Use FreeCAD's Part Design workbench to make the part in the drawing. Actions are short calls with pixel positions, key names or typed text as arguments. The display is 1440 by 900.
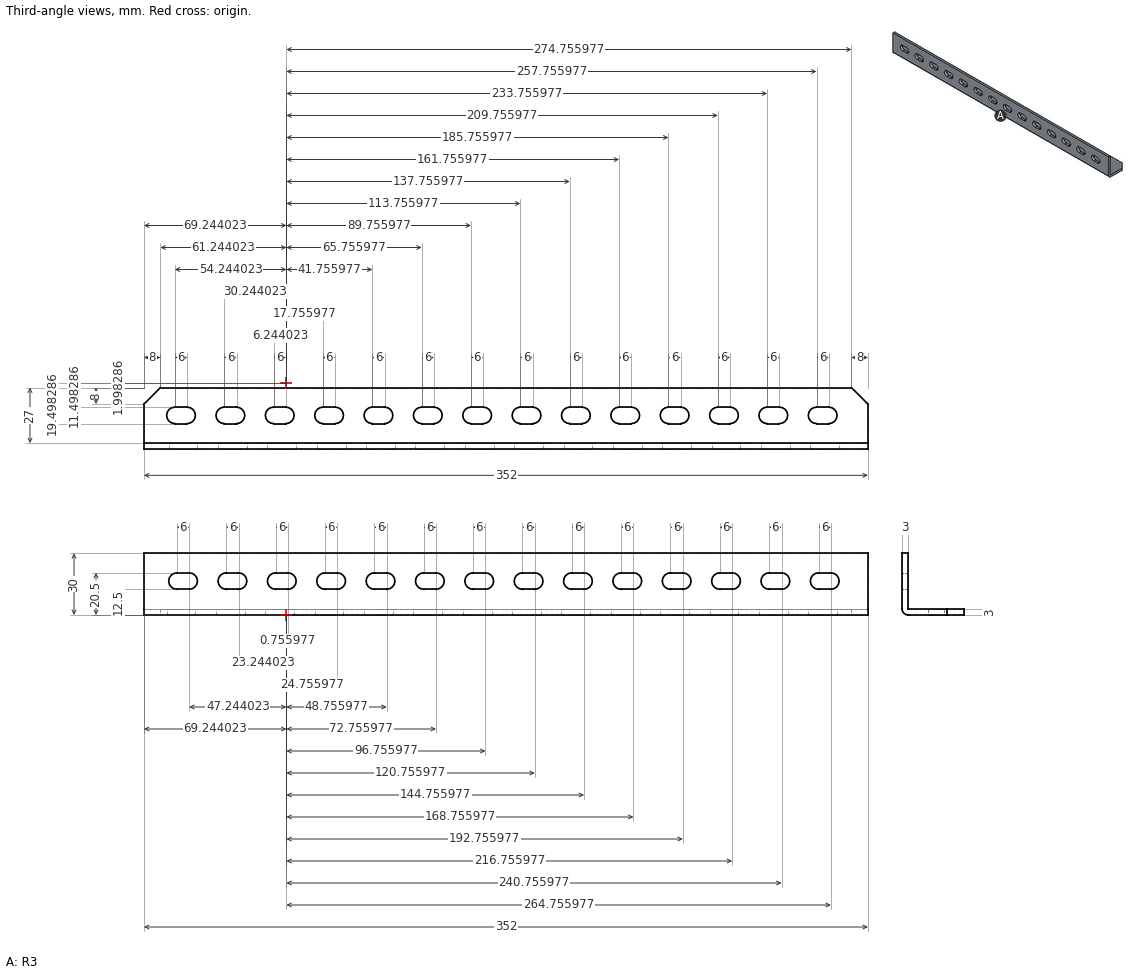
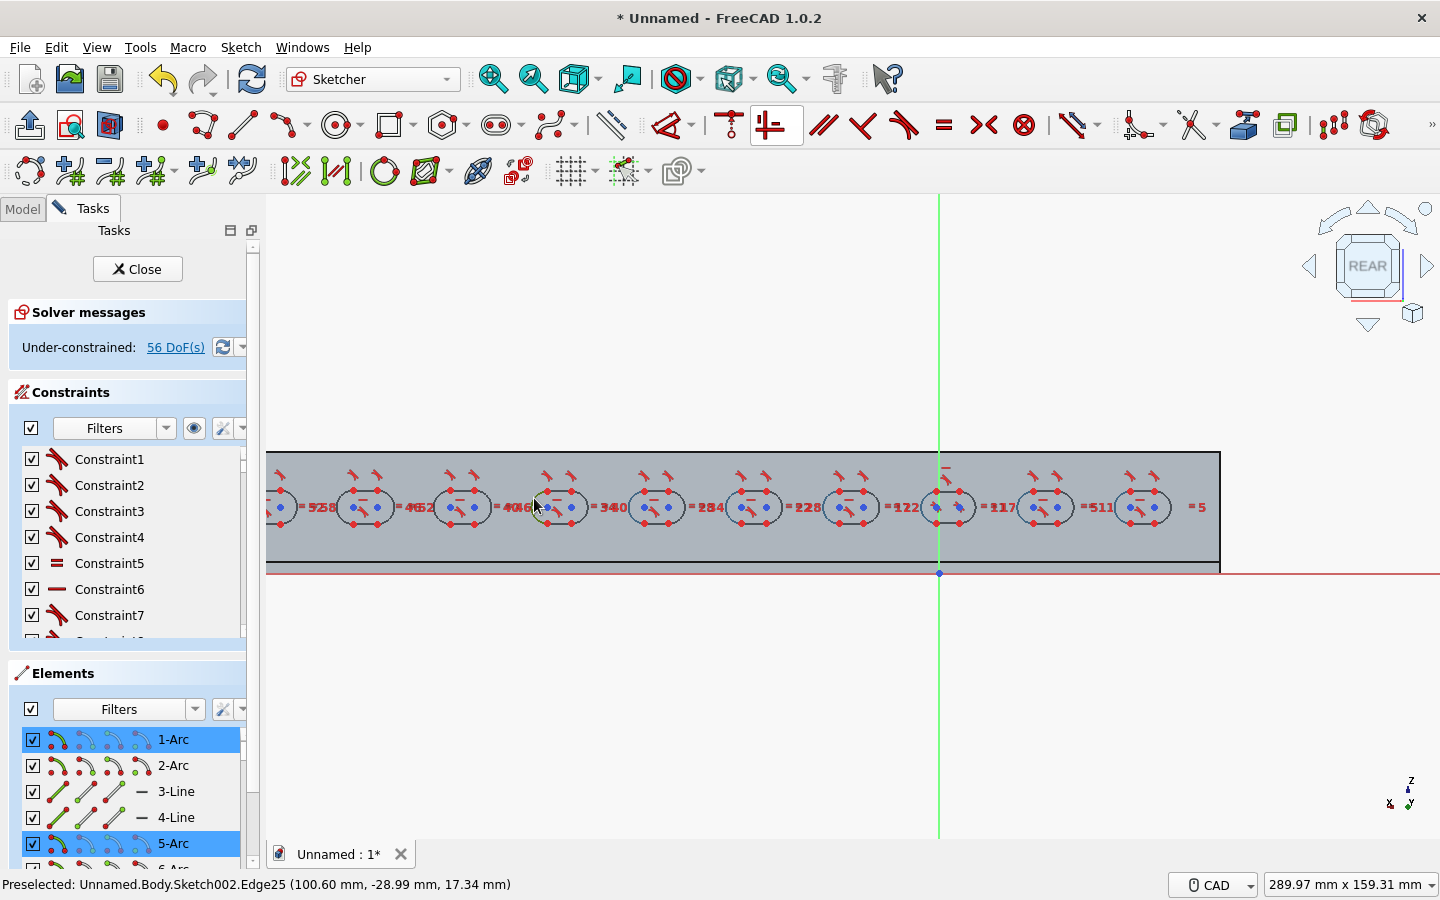
click(437, 497)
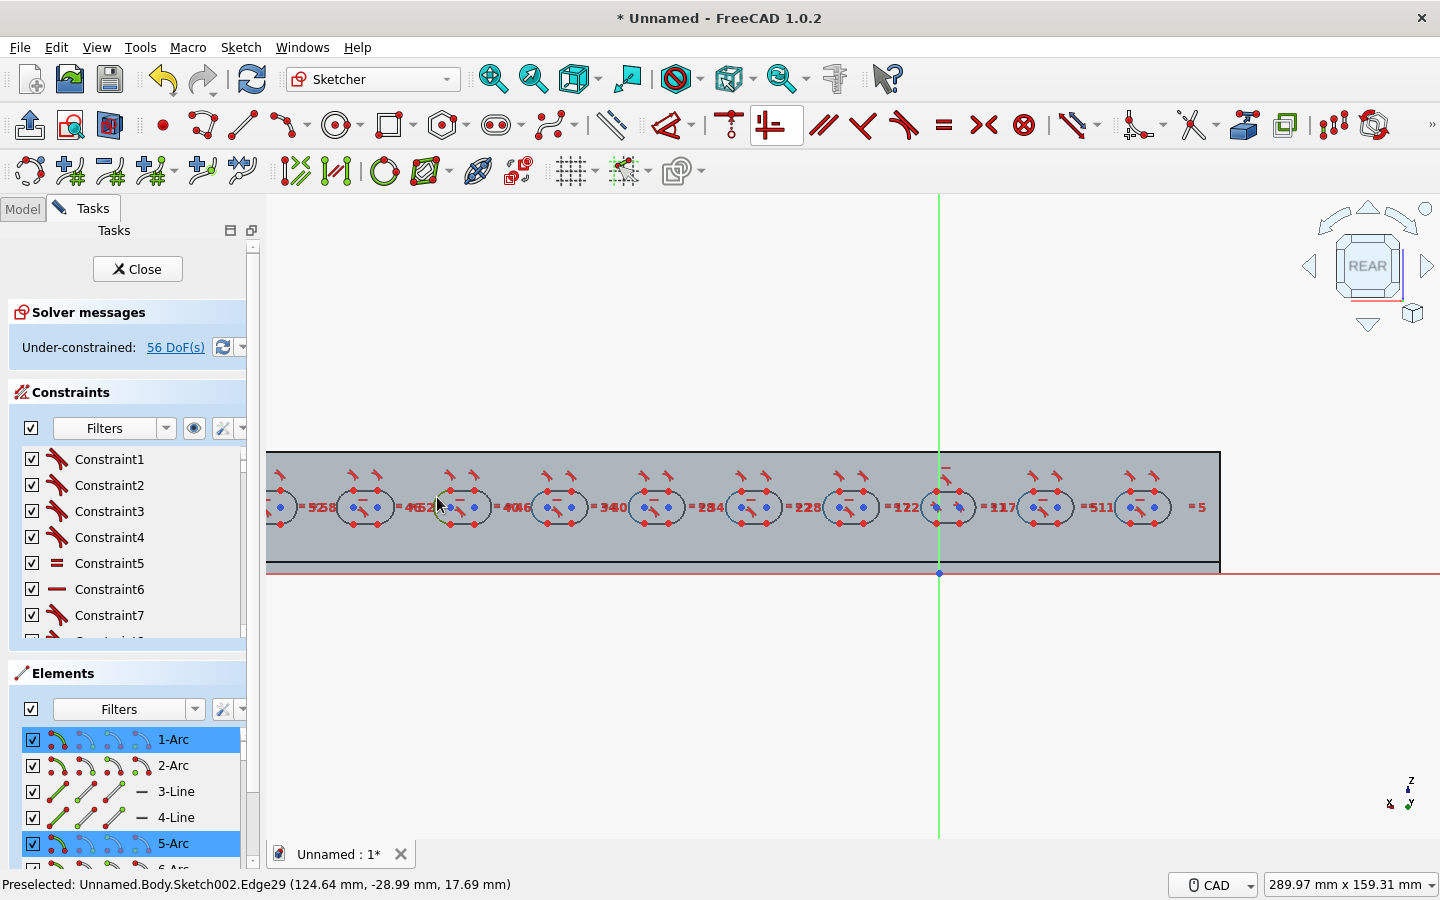
click(340, 497)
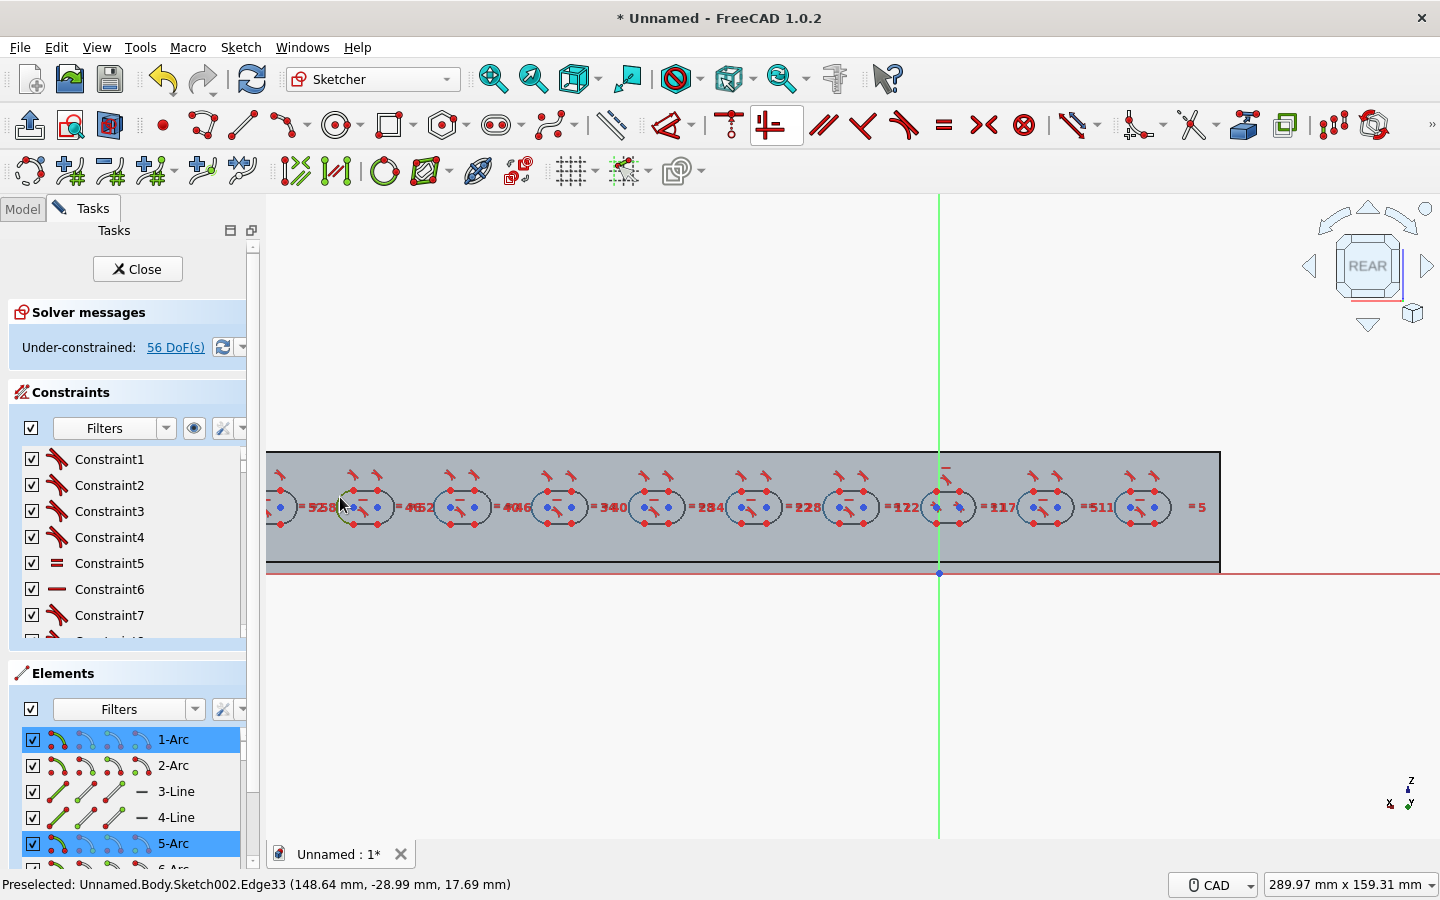
scroll(1117, 497, down, 3)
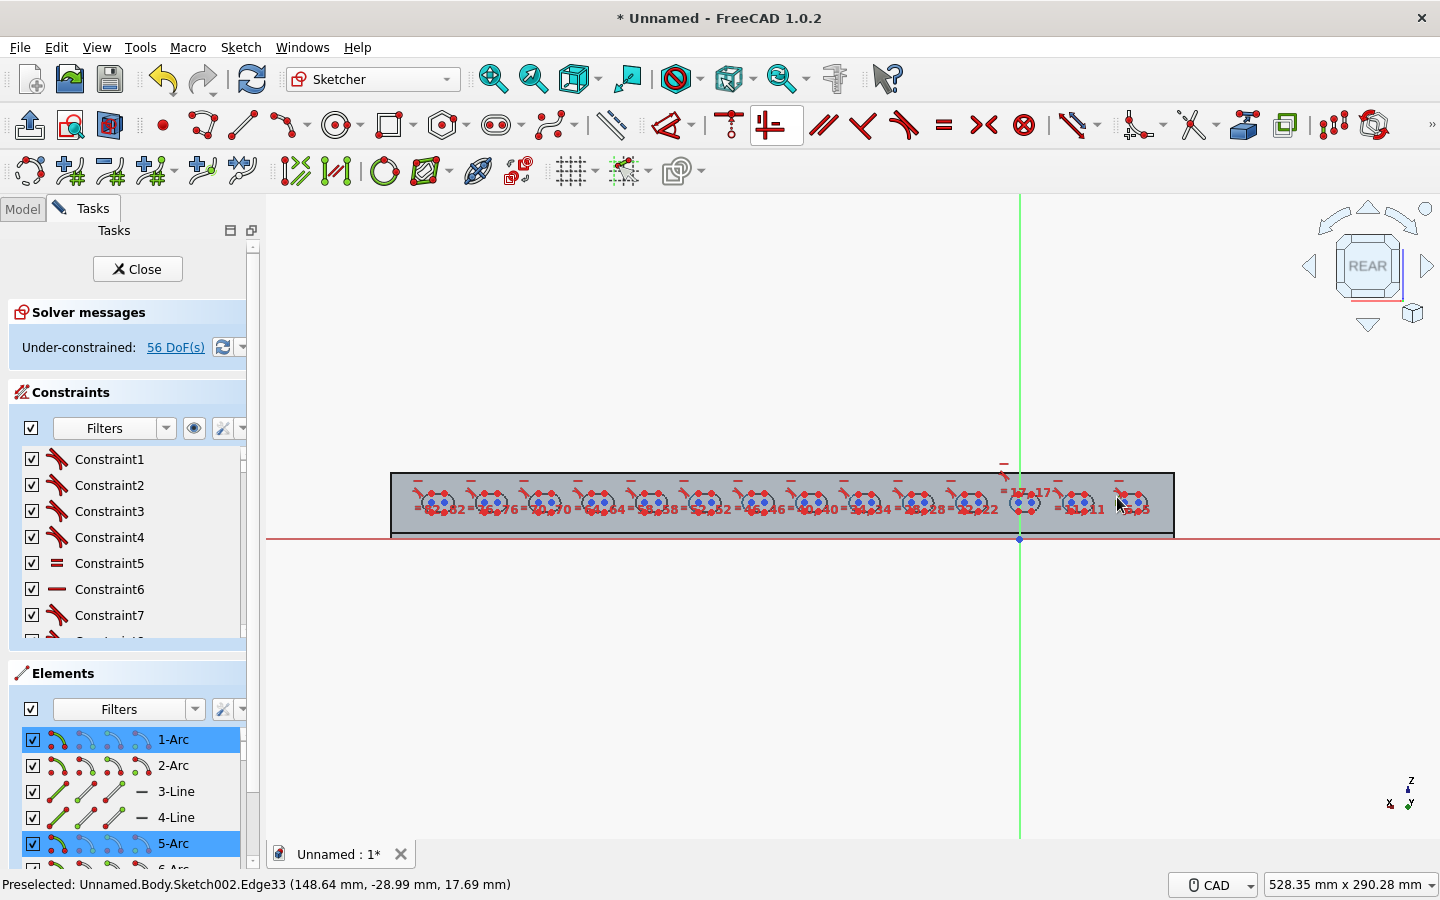
scroll(637, 497, up, 3)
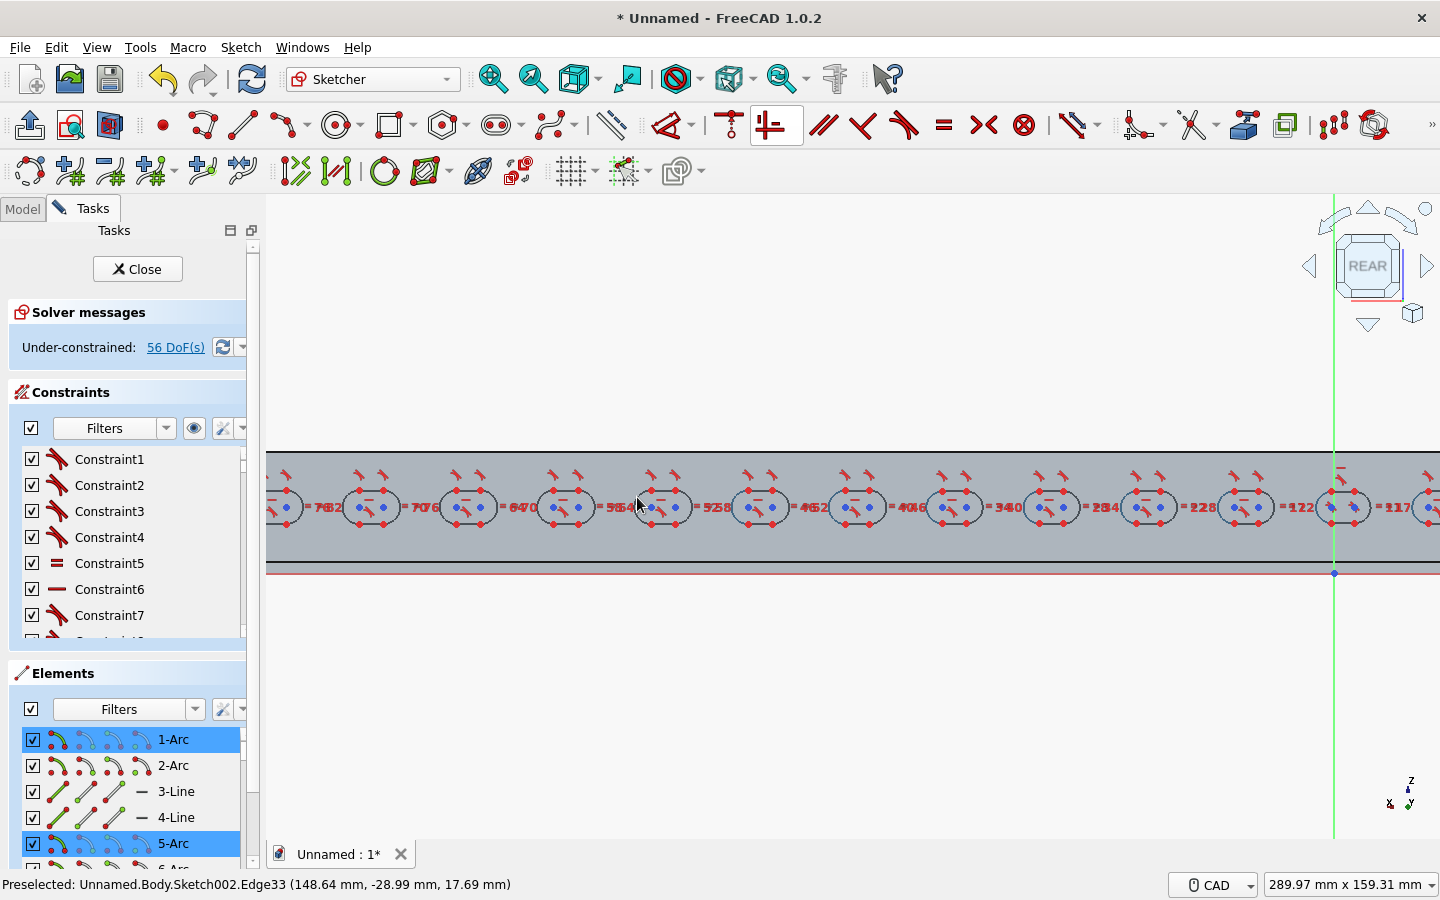
click(638, 497)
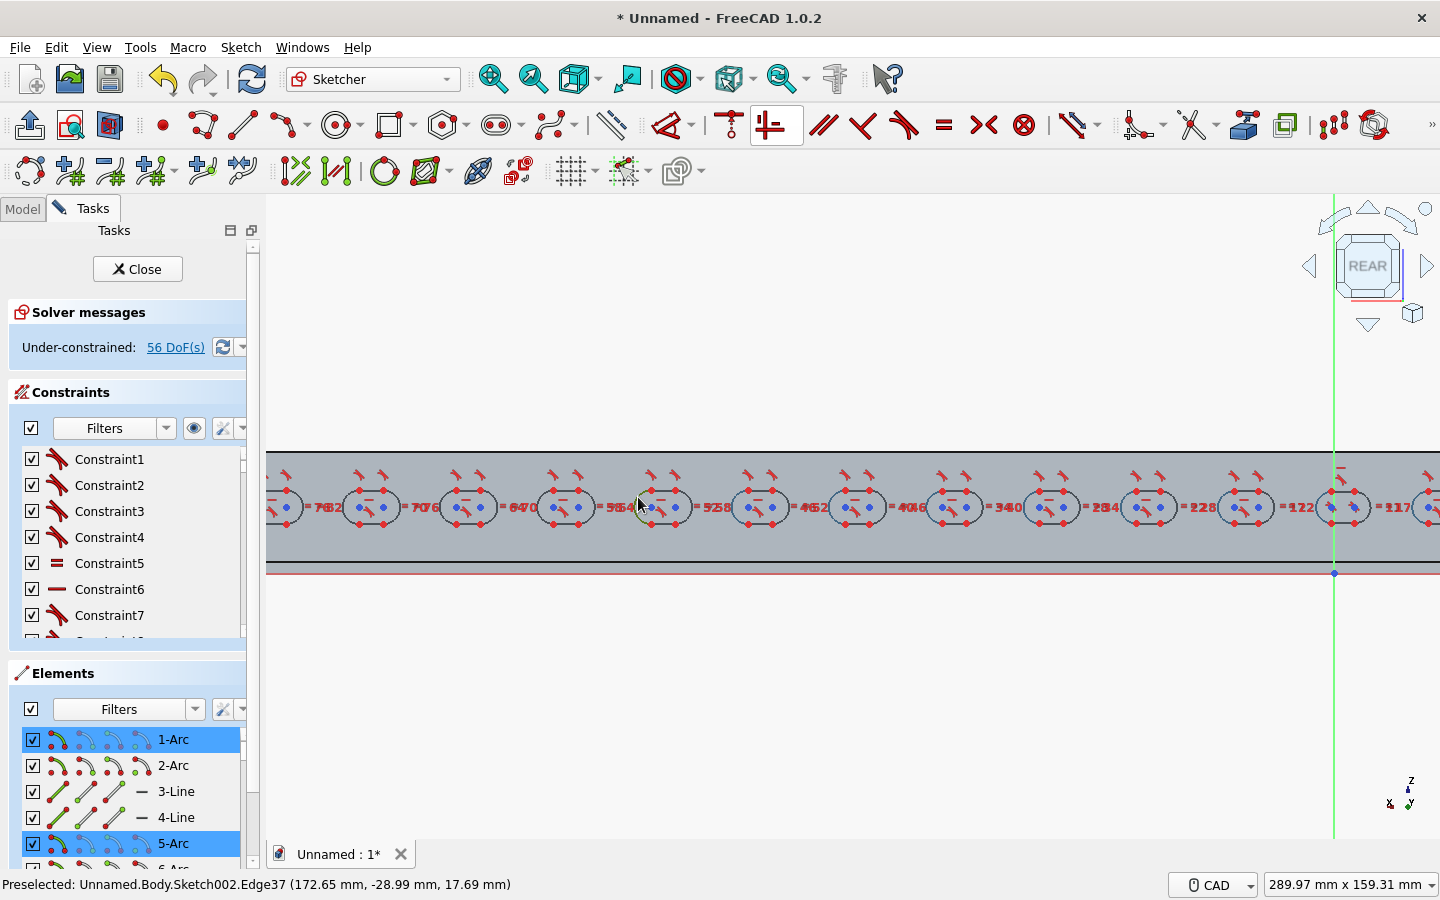
click(540, 497)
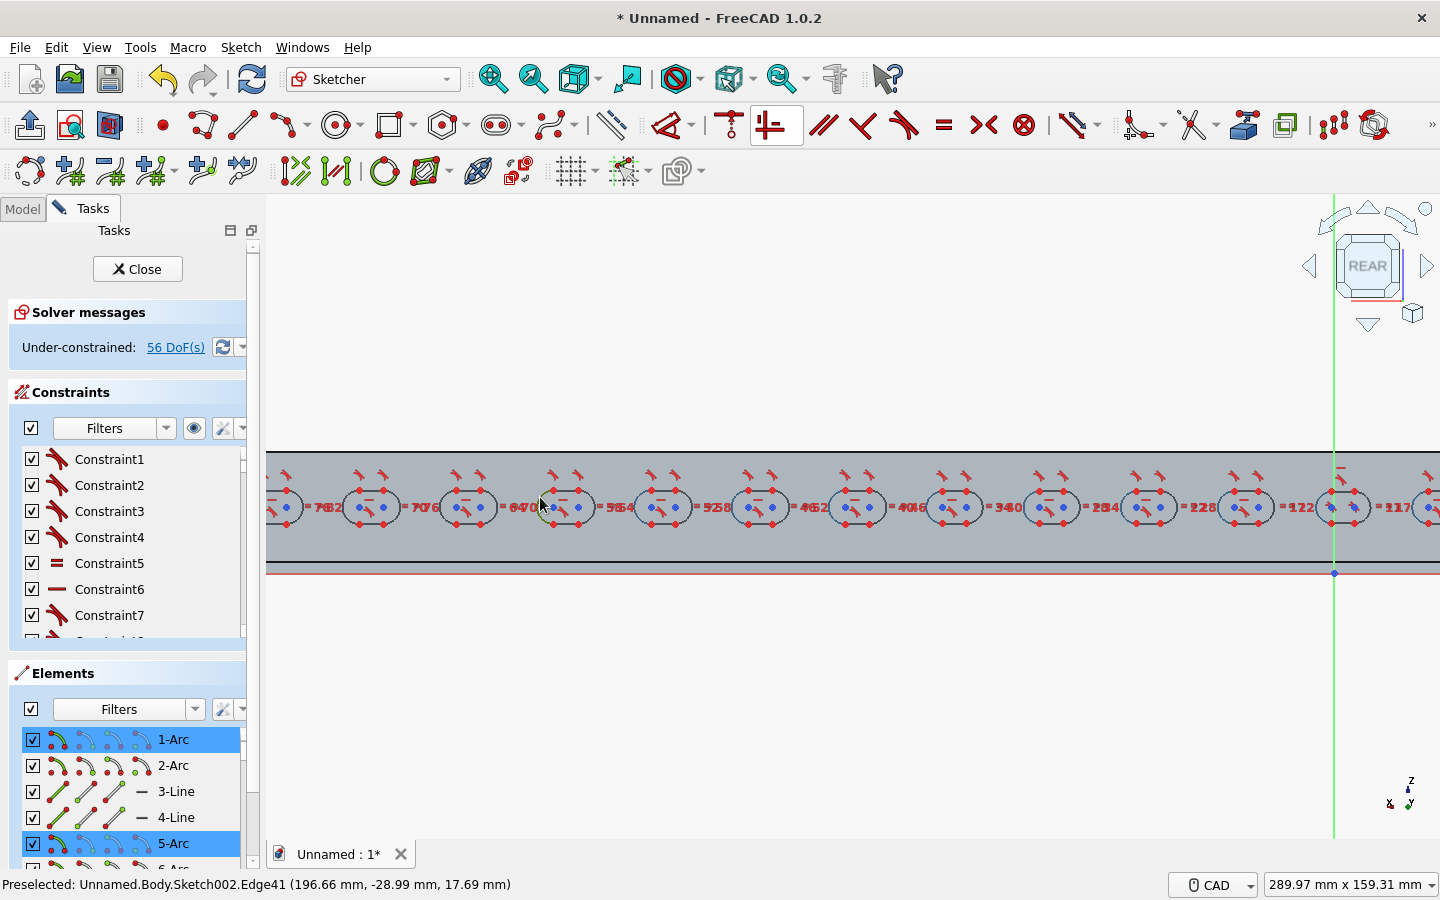
click(443, 497)